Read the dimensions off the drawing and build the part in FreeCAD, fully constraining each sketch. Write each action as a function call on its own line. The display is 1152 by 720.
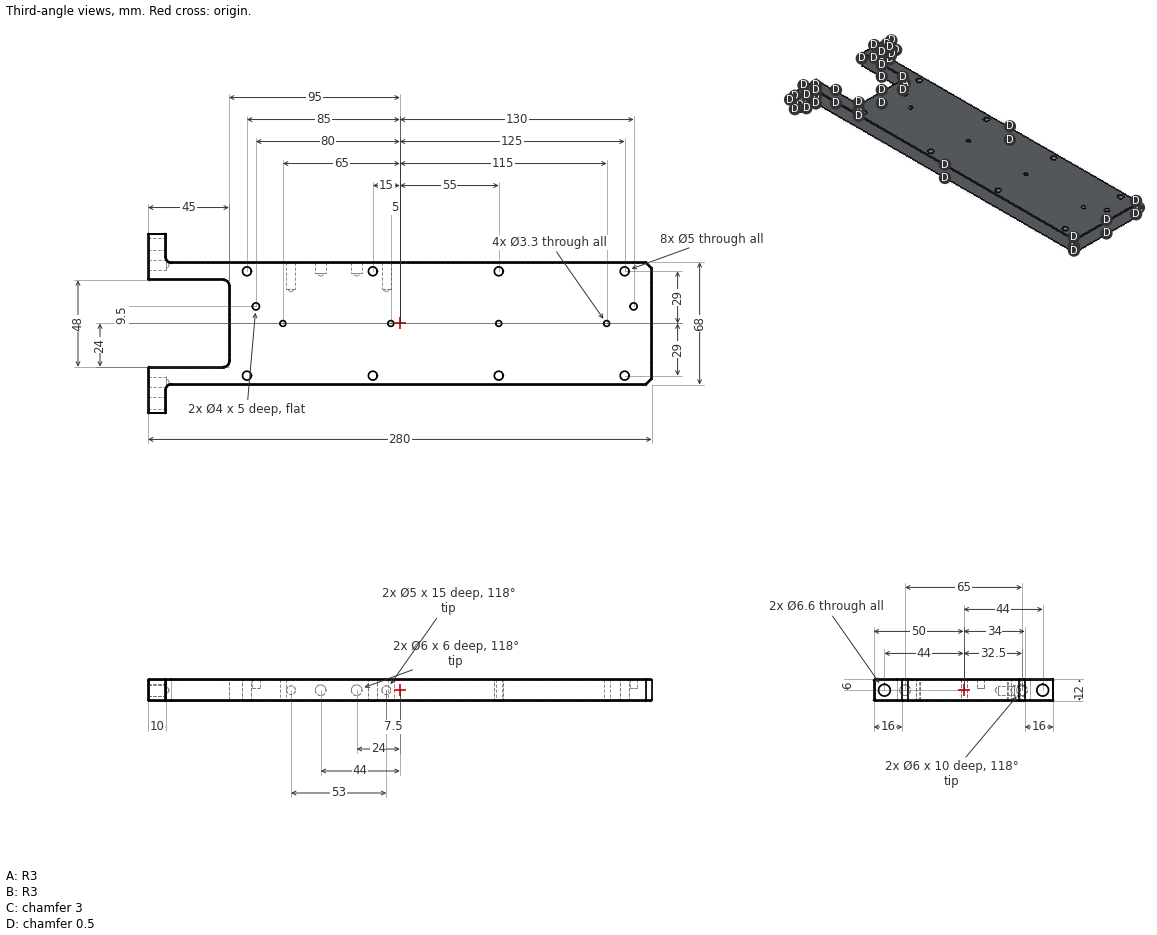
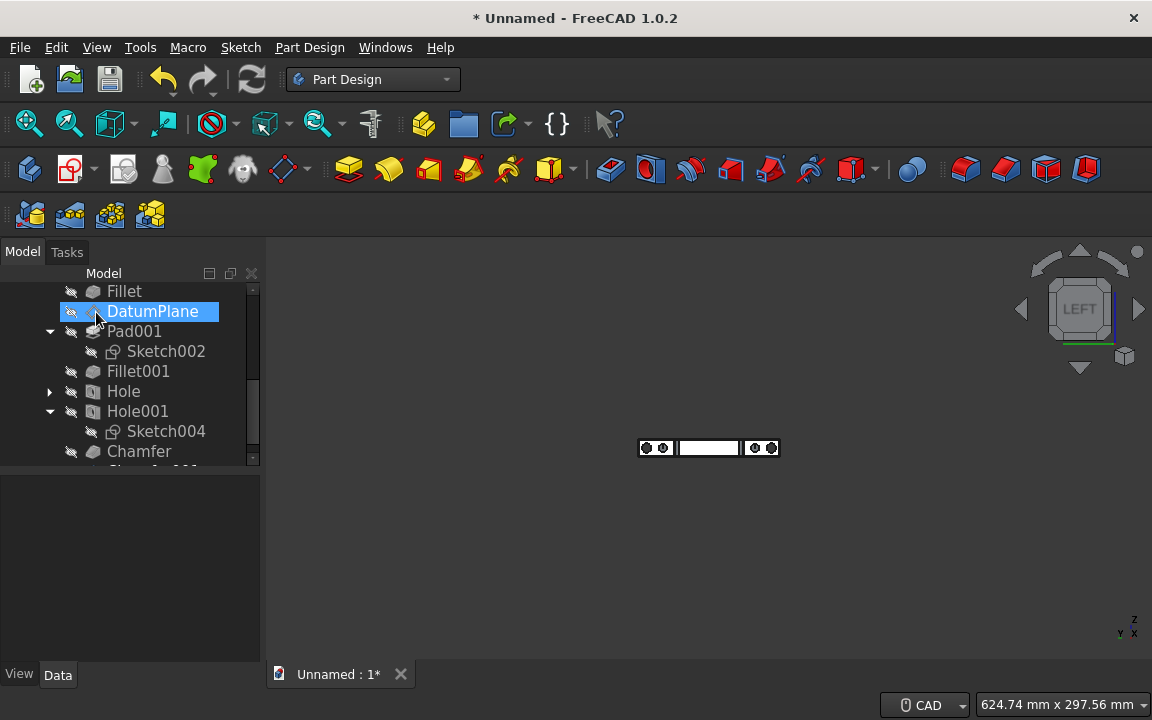
key(5)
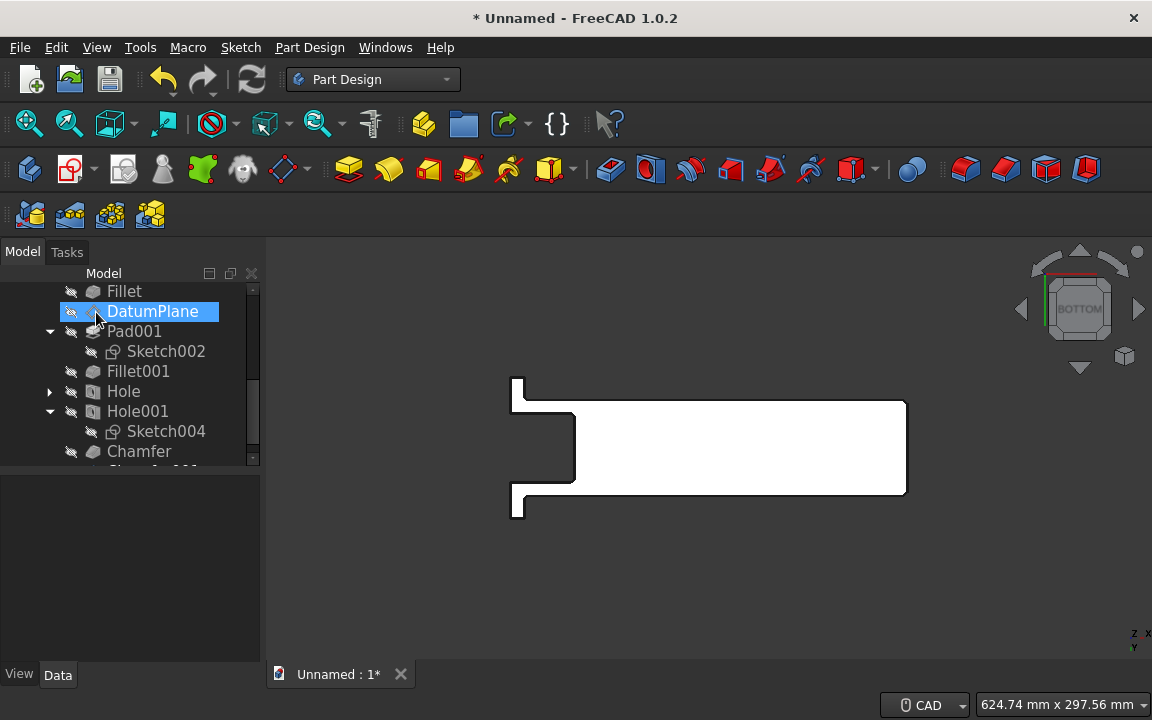
key(v)
key(f)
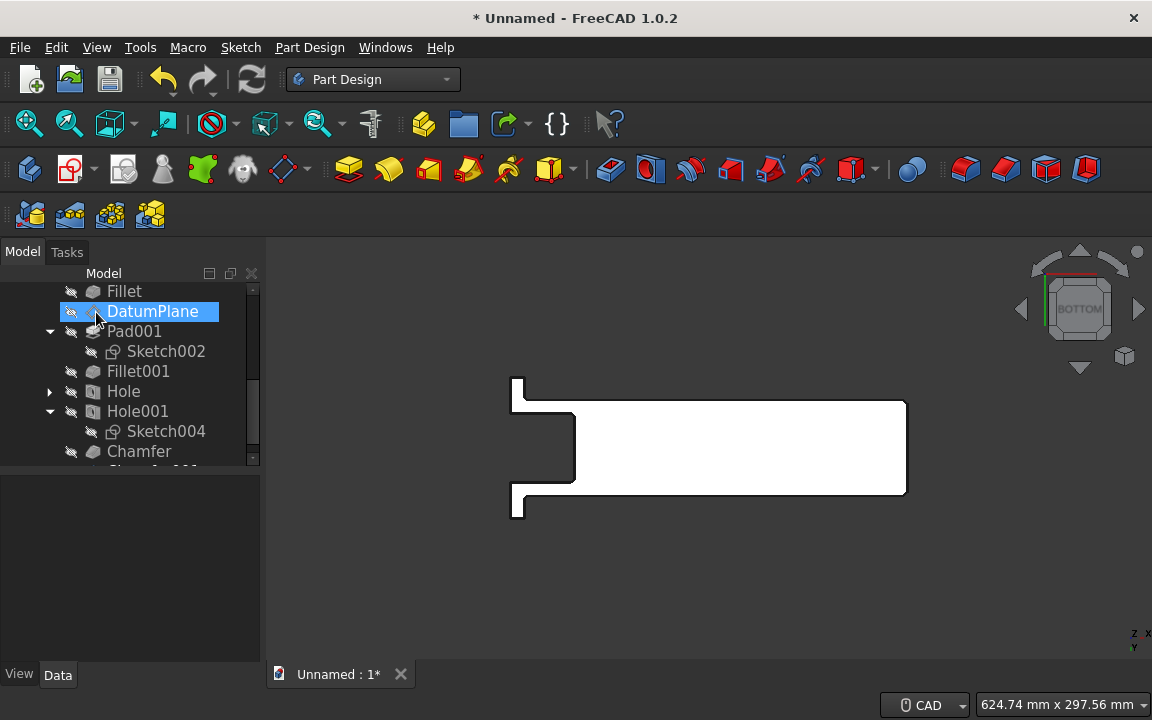
click(822, 447)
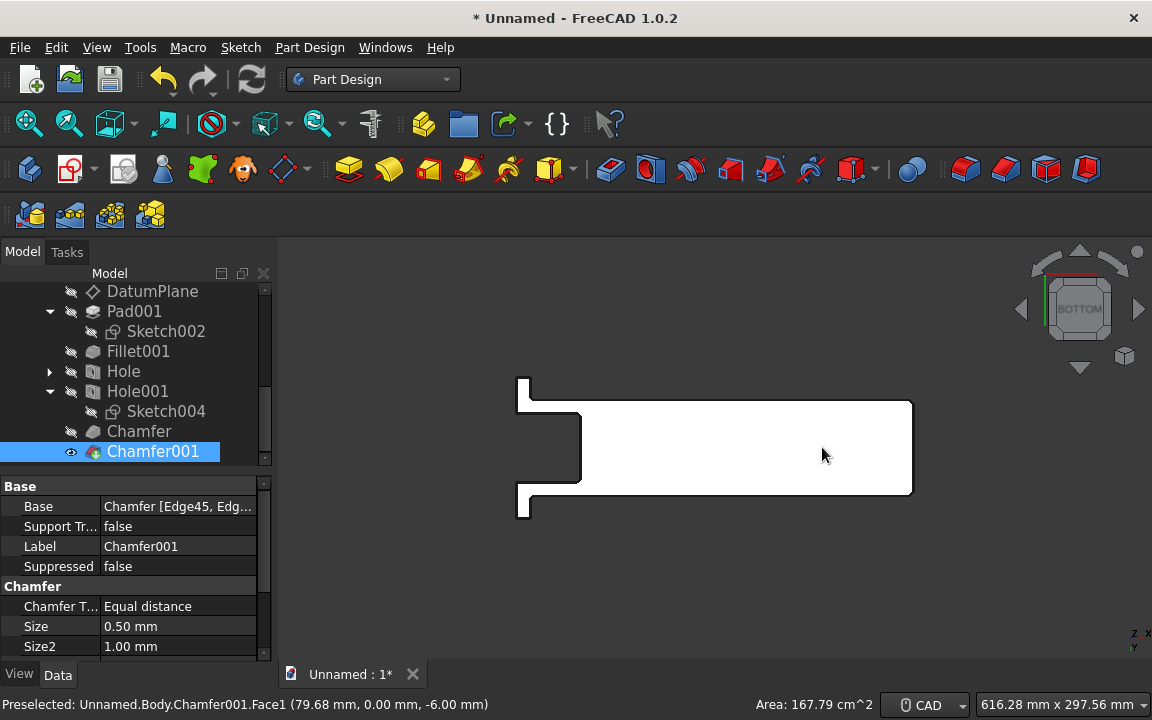
click(70, 170)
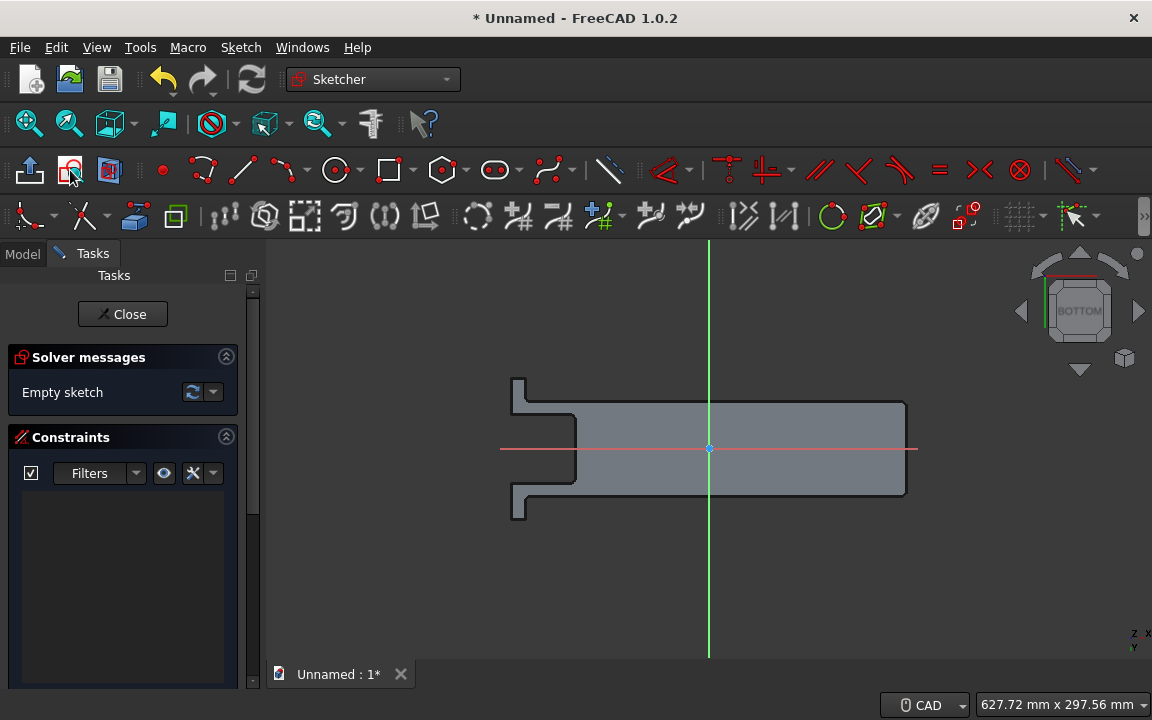
scroll(934, 449, up, 2)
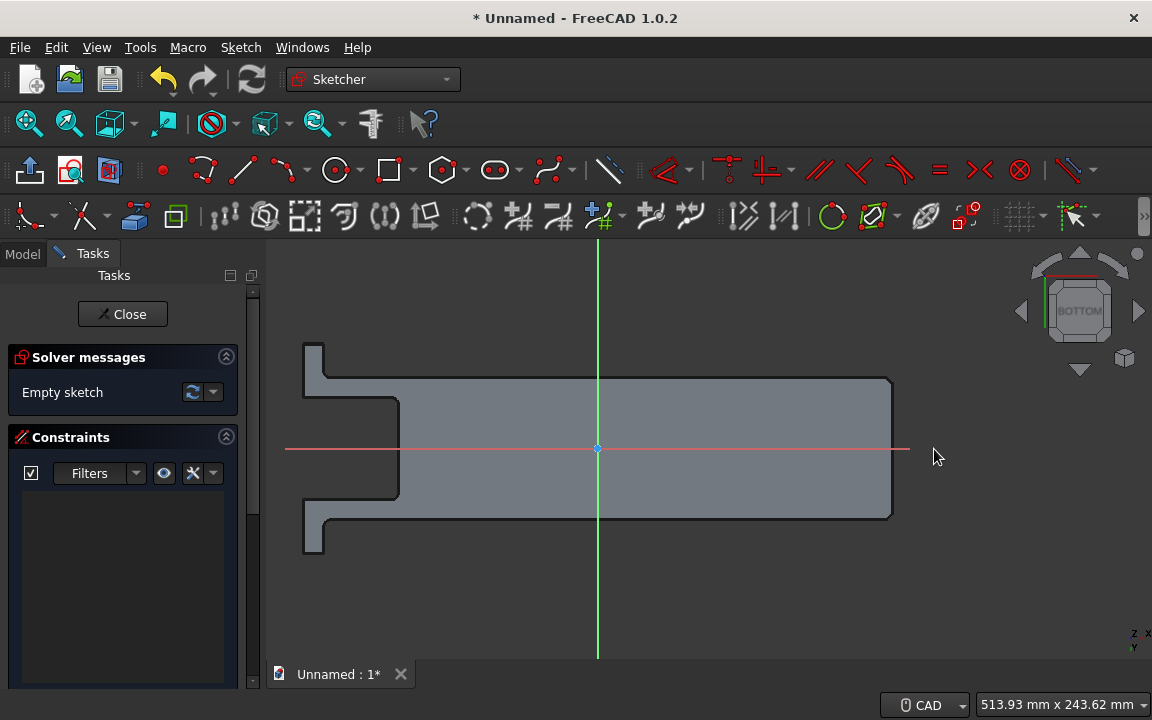
click(336, 170)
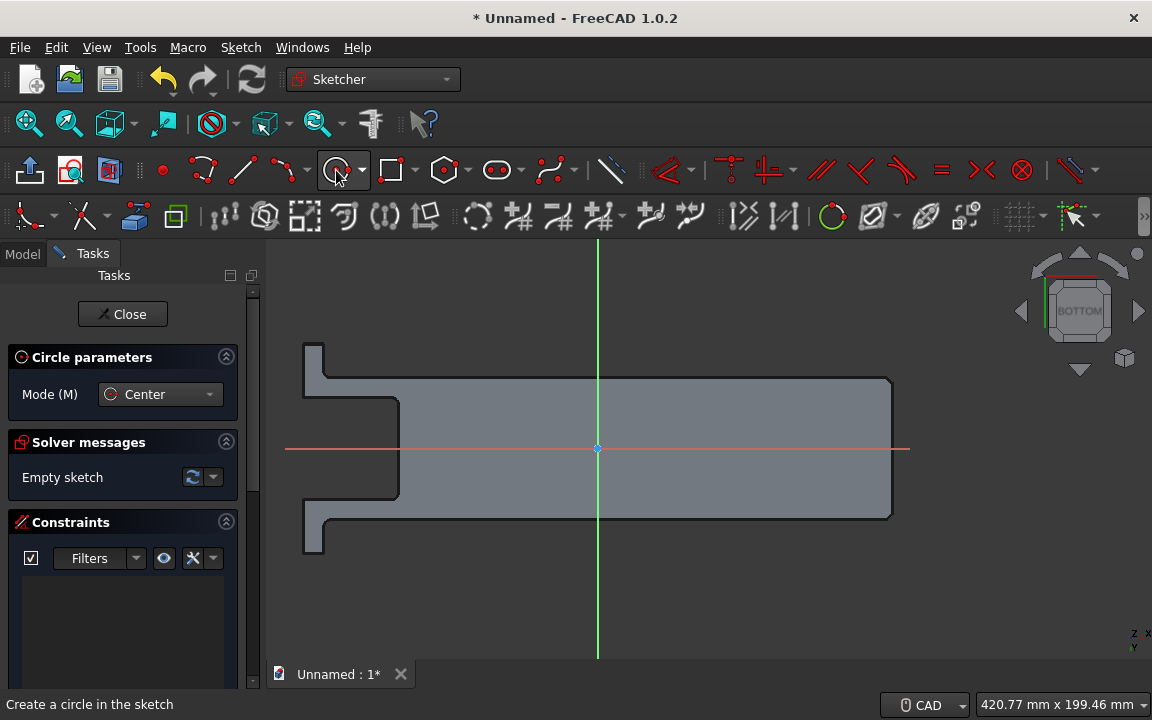
scroll(861, 510, up, 8)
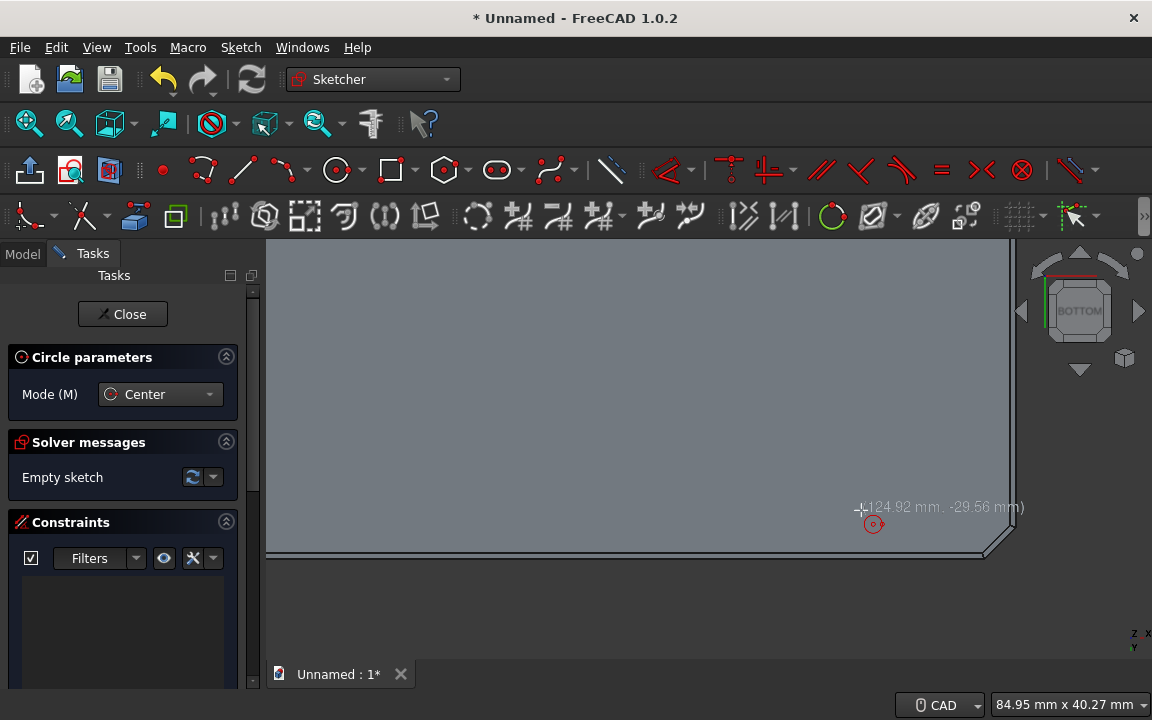
scroll(862, 511, down, 8)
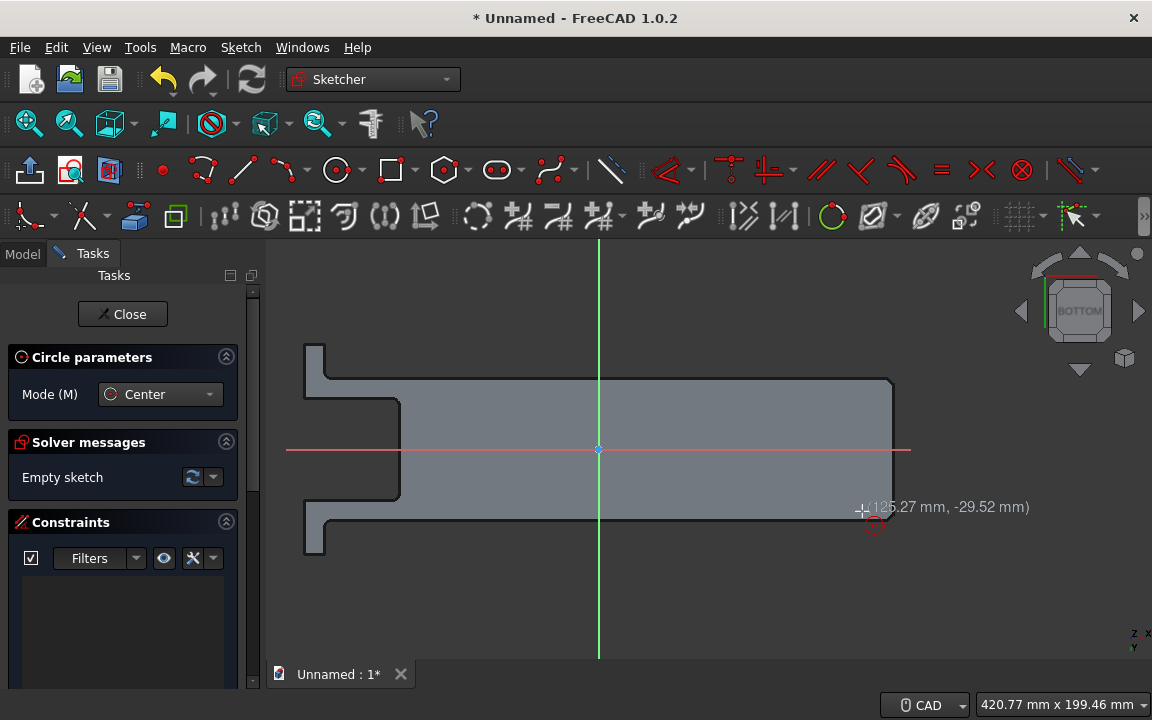
click(862, 511)
move(866, 507)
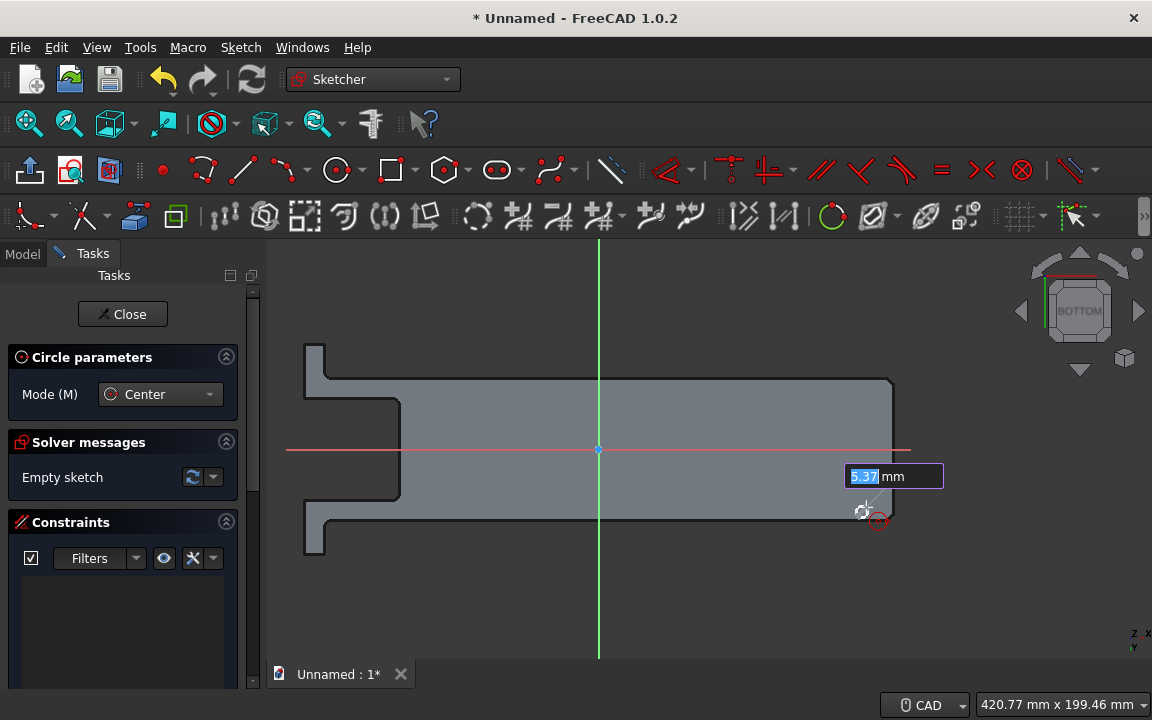
text(5)
key(Return)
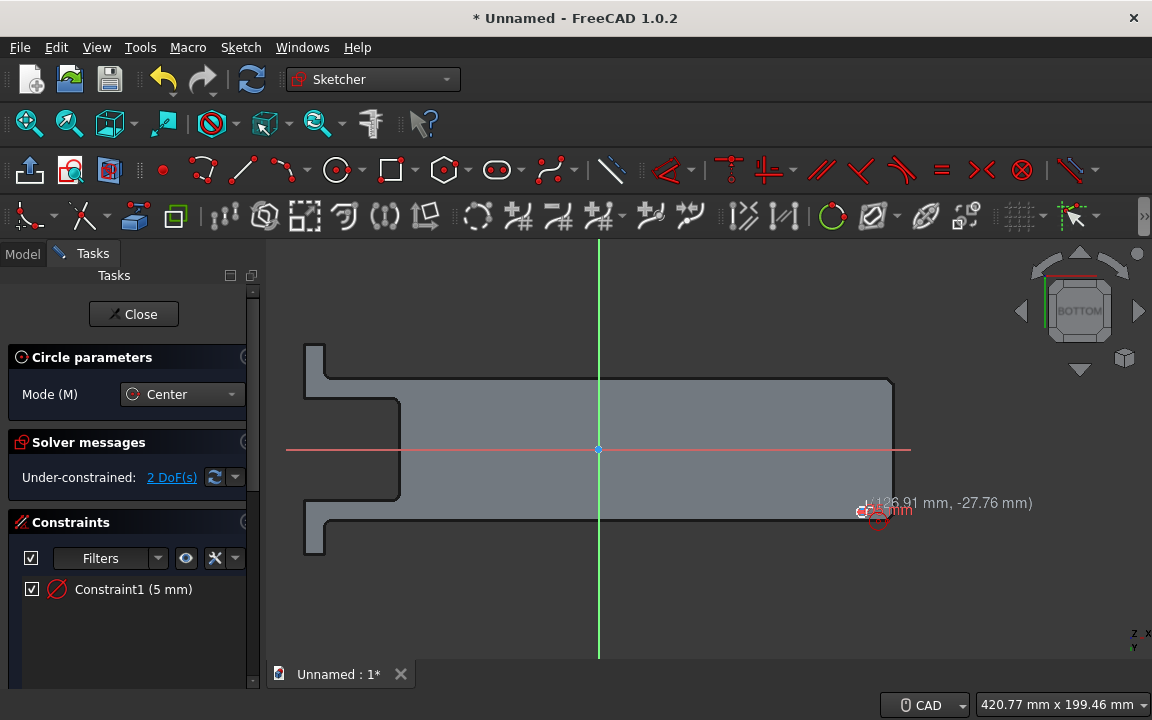
scroll(862, 388, up, 8)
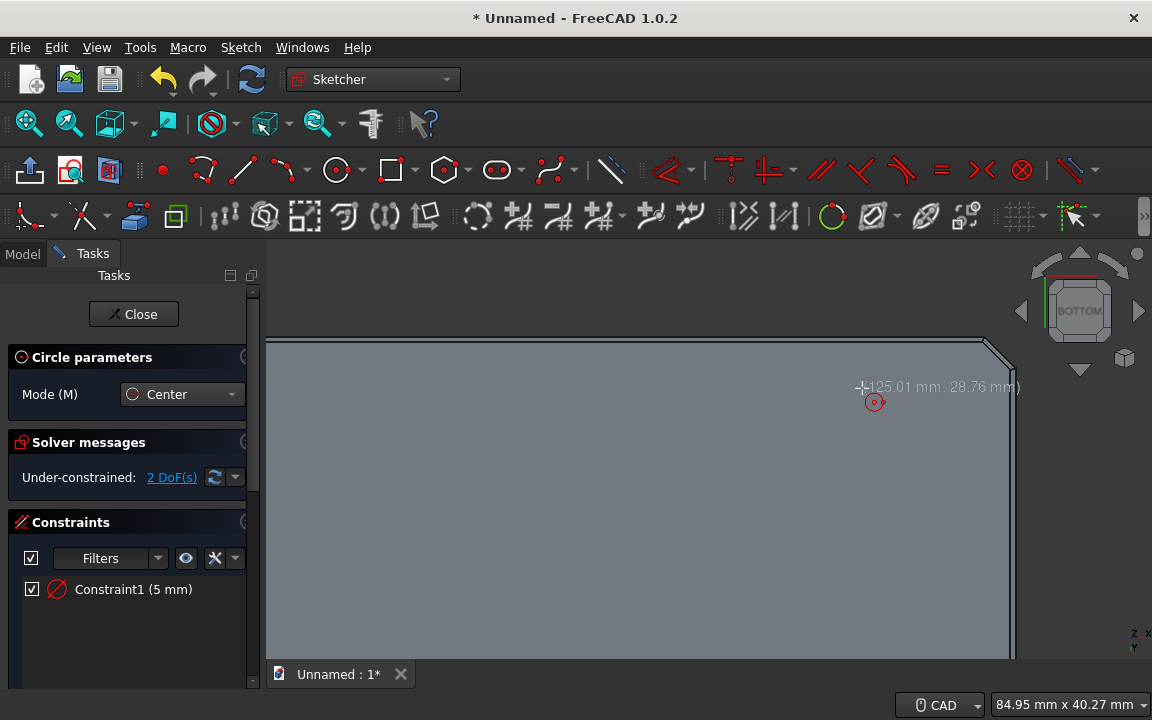
scroll(862, 388, down, 8)